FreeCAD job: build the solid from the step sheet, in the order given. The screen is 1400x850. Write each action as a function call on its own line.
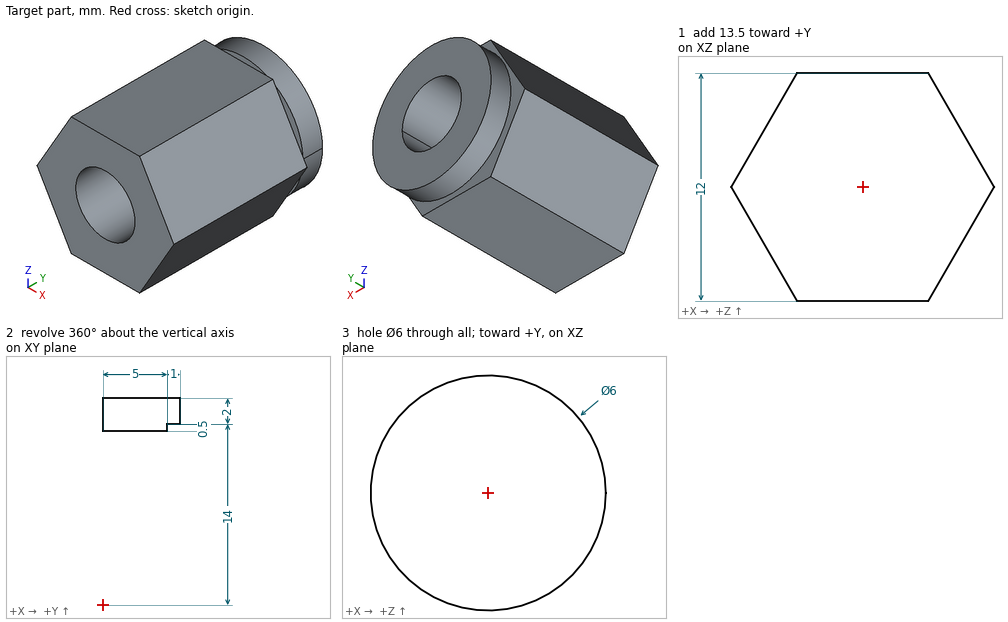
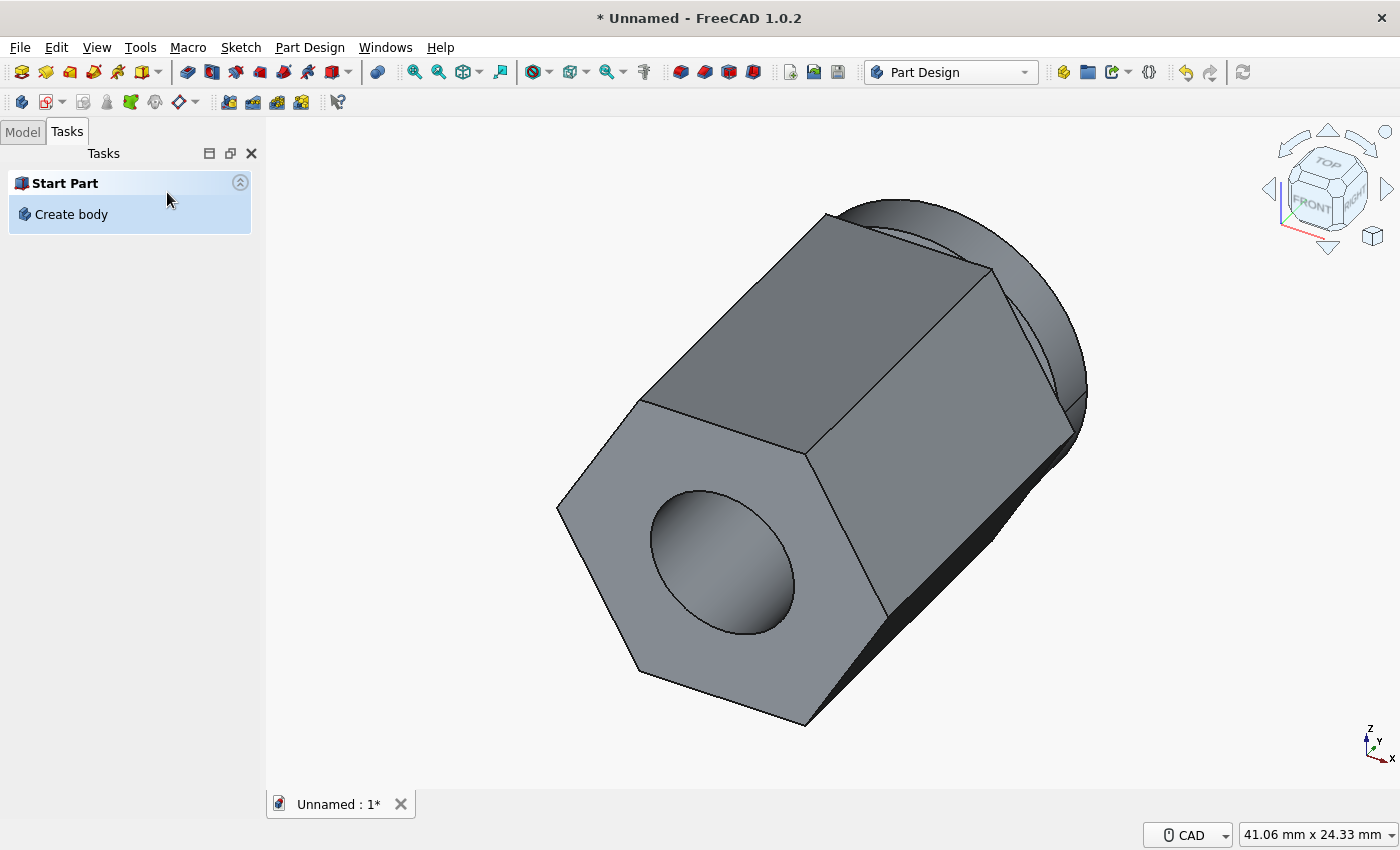
key(0)